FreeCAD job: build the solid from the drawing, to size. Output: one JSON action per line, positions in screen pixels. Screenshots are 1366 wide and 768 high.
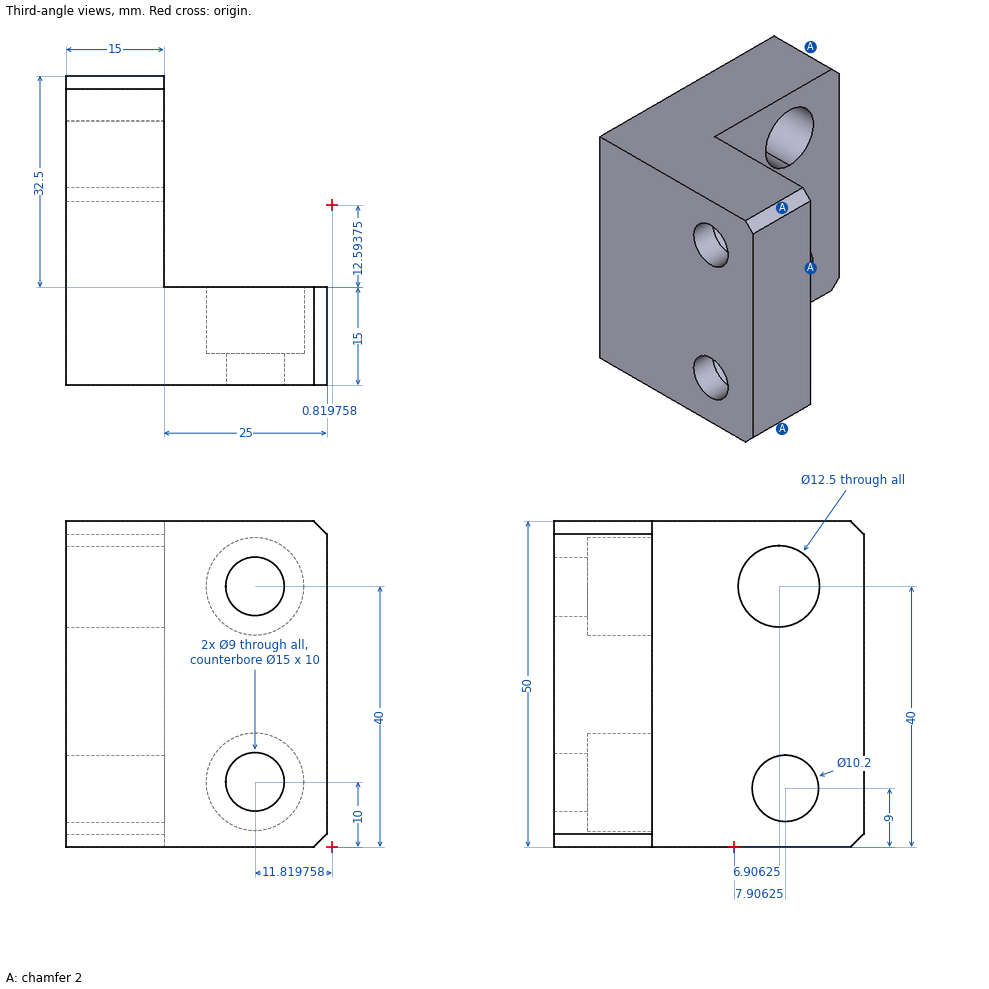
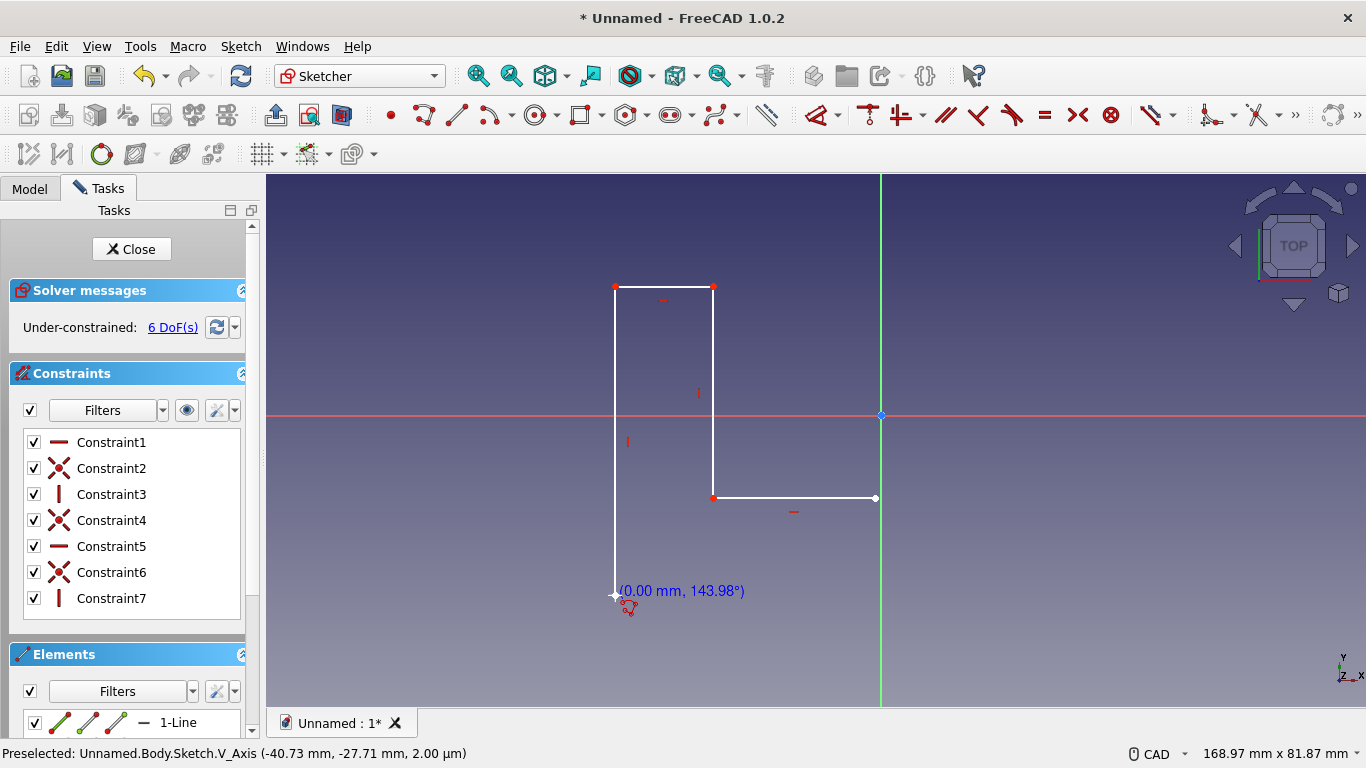
{"action": "scroll", "coordinate": [876, 595], "scroll_direction": "up", "scroll_amount": 6}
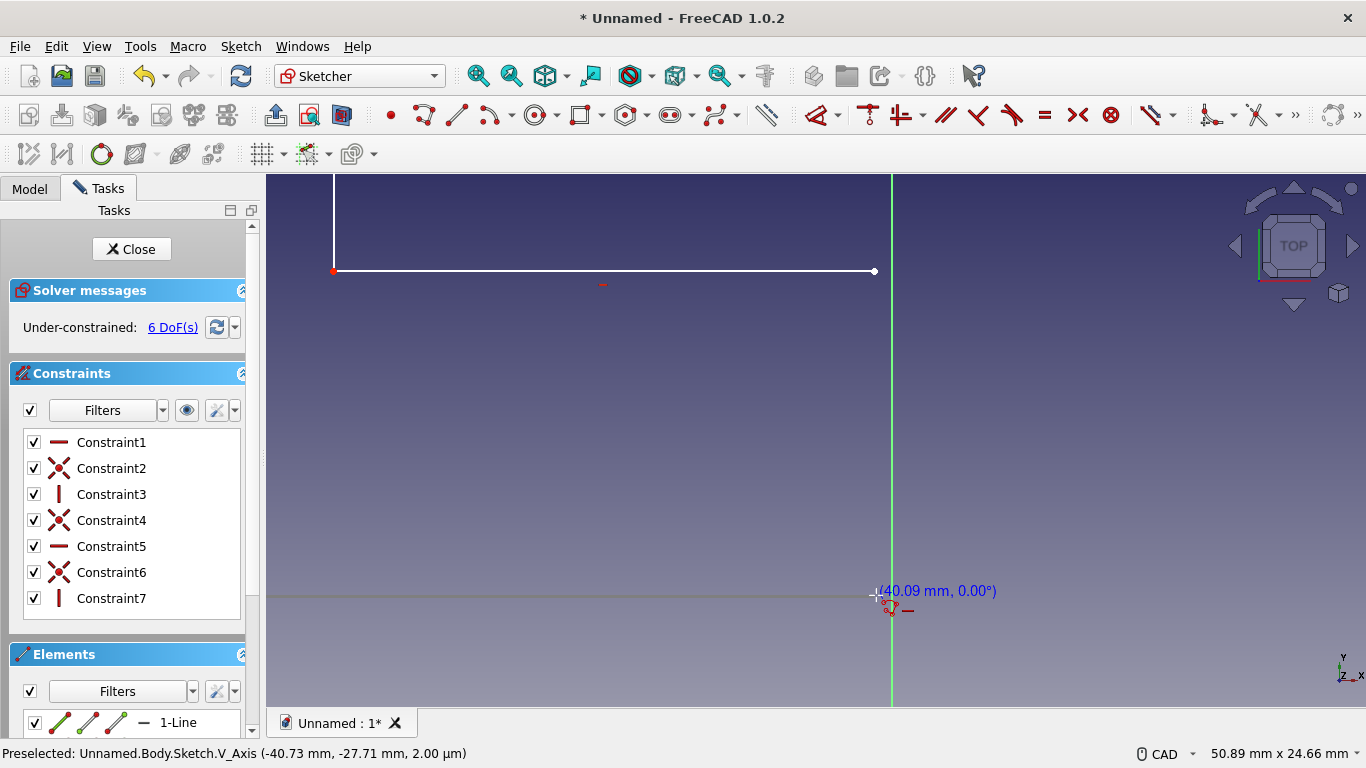
{"action": "left_click", "coordinate": [874, 593]}
{"action": "left_click", "coordinate": [874, 271]}
{"action": "key", "text": "Escape"}
{"action": "key", "text": "Escape"}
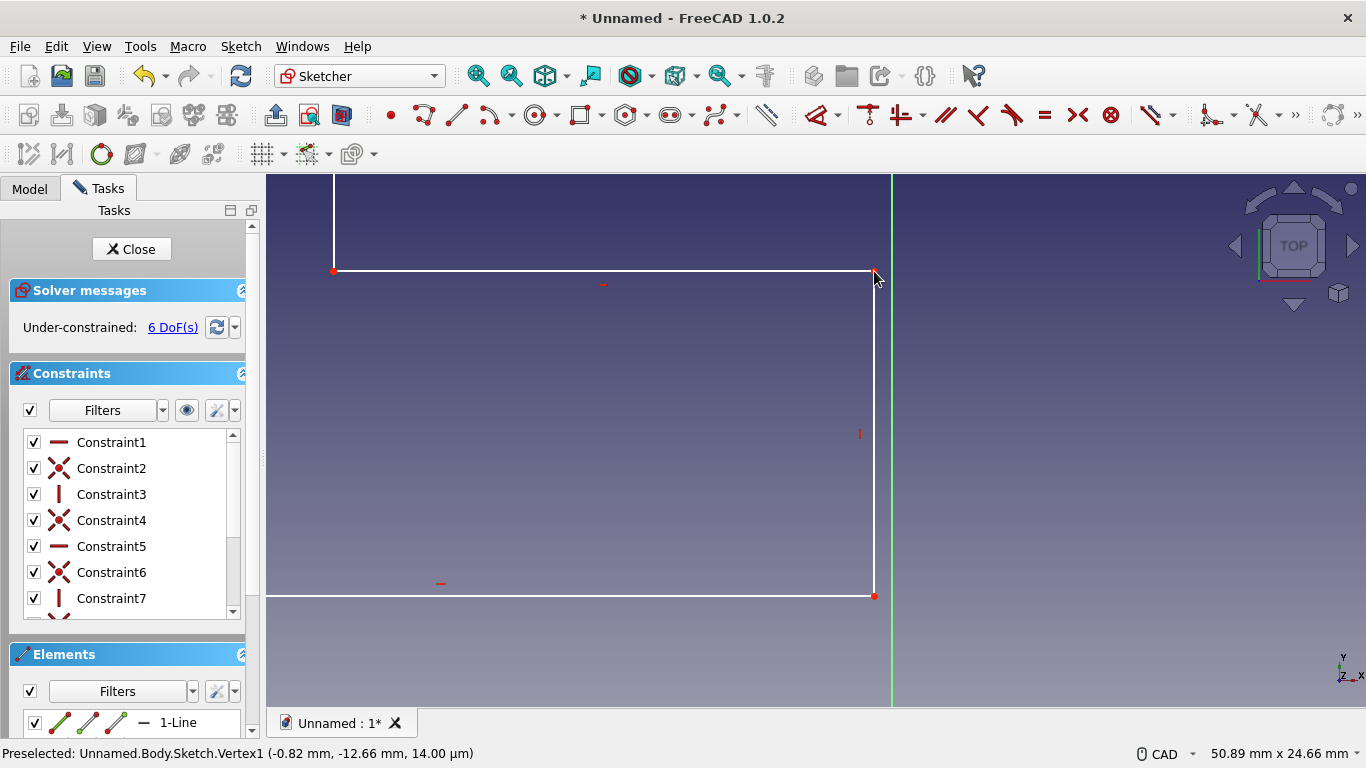
{"action": "left_click", "coordinate": [816, 116]}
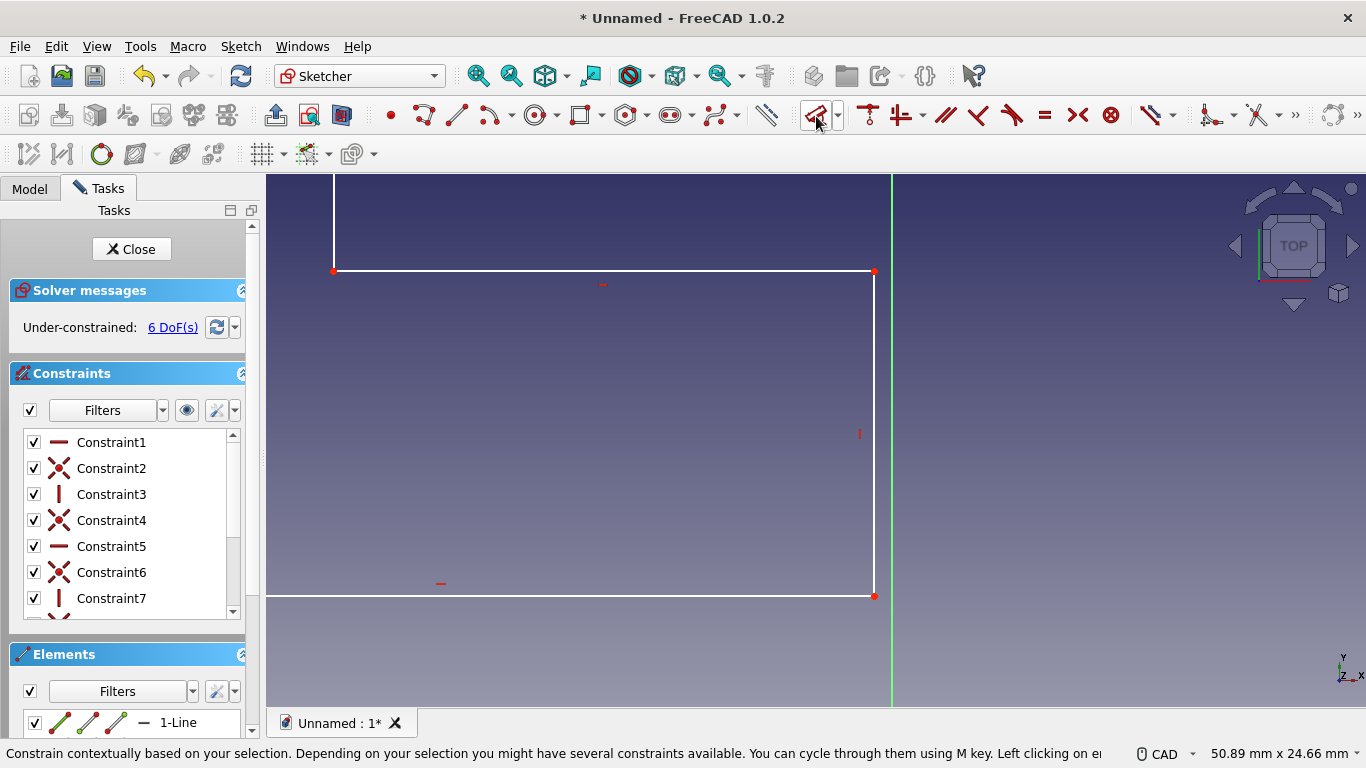
{"action": "scroll", "coordinate": [875, 596], "scroll_direction": "down", "scroll_amount": 6}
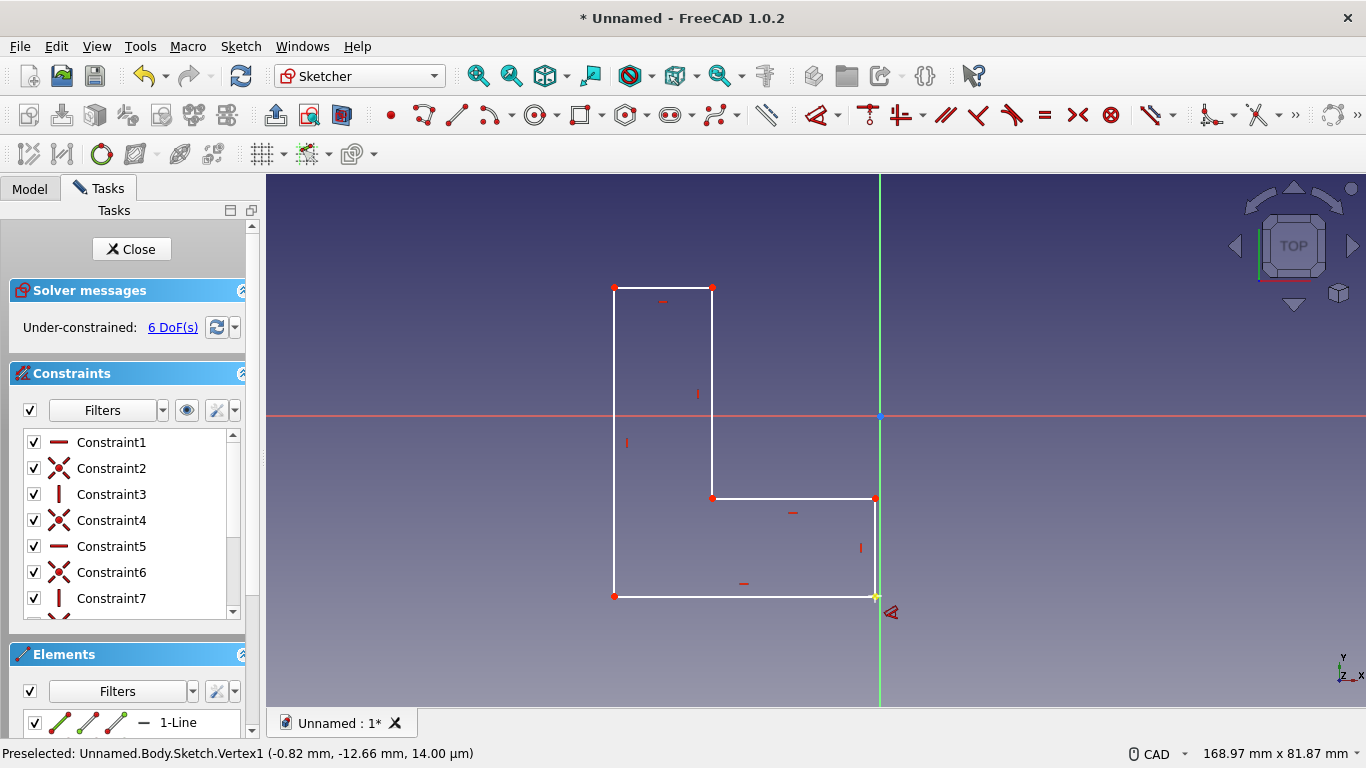
{"action": "left_click", "coordinate": [826, 499]}
{"action": "left_click", "coordinate": [794, 533]}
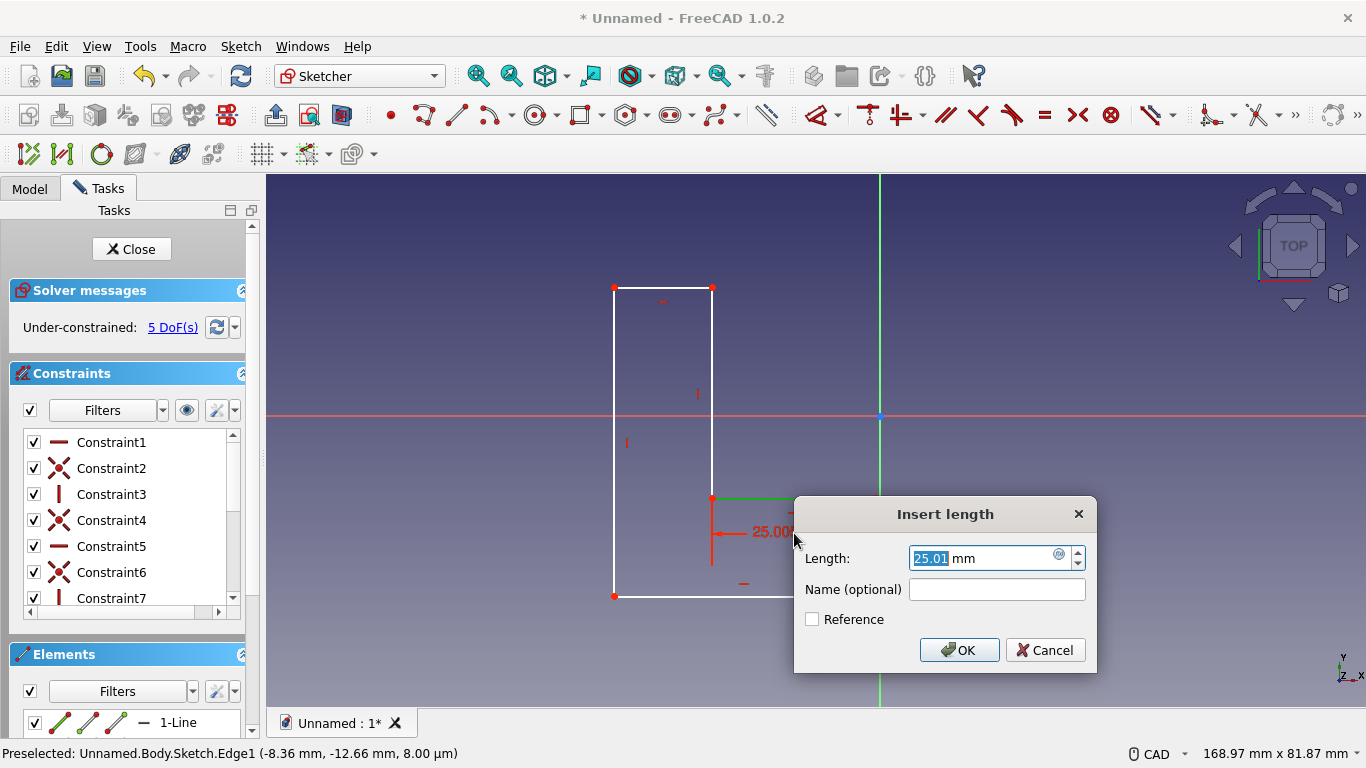
{"action": "type", "text": "25"}
{"action": "key", "text": "Return"}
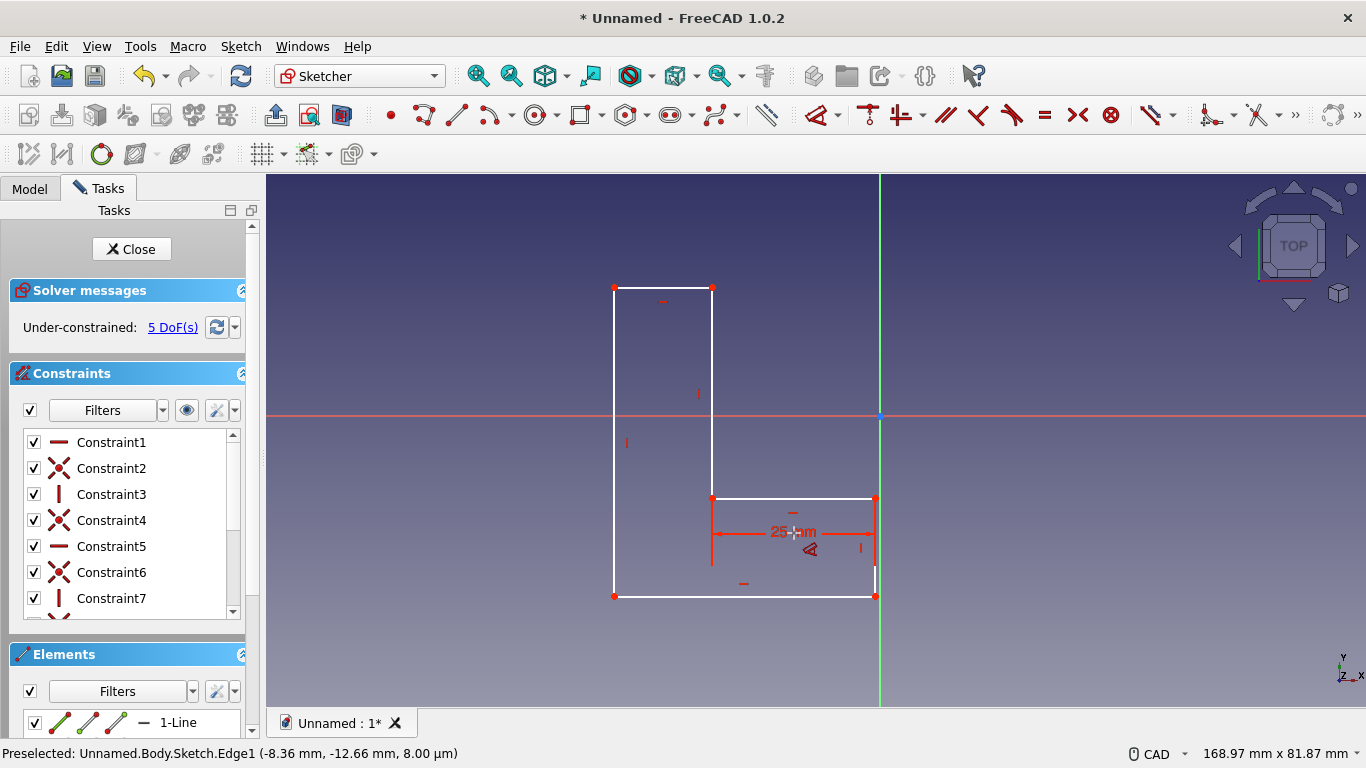
{"action": "left_click", "coordinate": [683, 288]}
{"action": "left_click", "coordinate": [663, 254]}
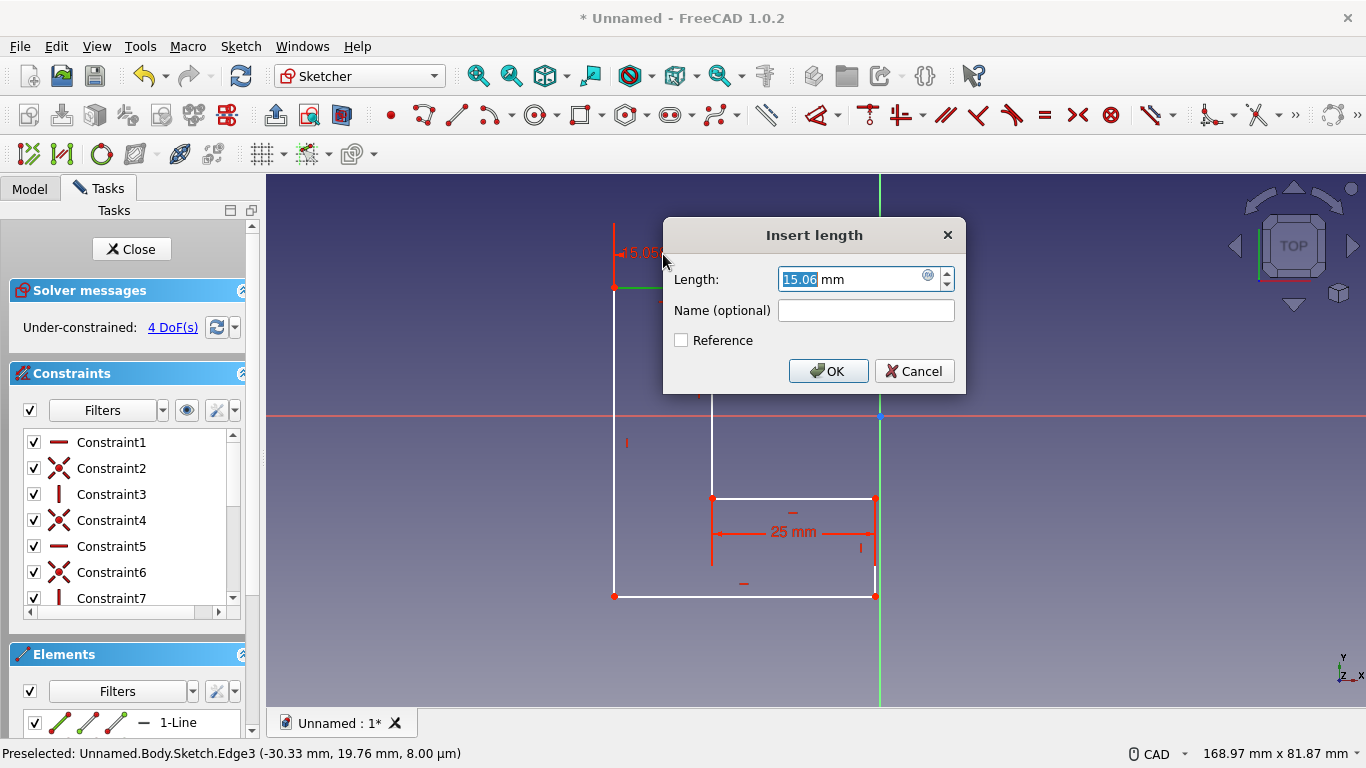
{"action": "type", "text": "15"}
{"action": "key", "text": "Return"}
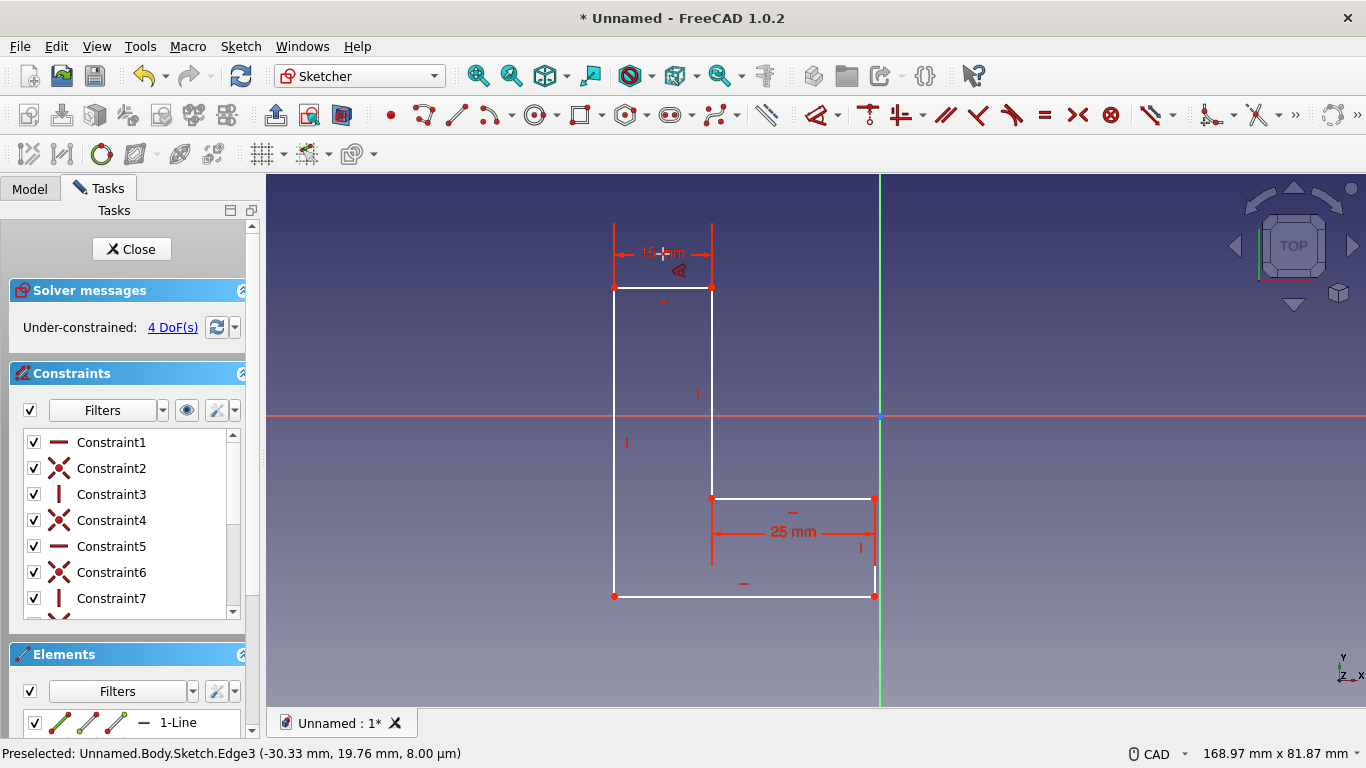
{"action": "scroll", "coordinate": [875, 567], "scroll_direction": "up", "scroll_amount": 5}